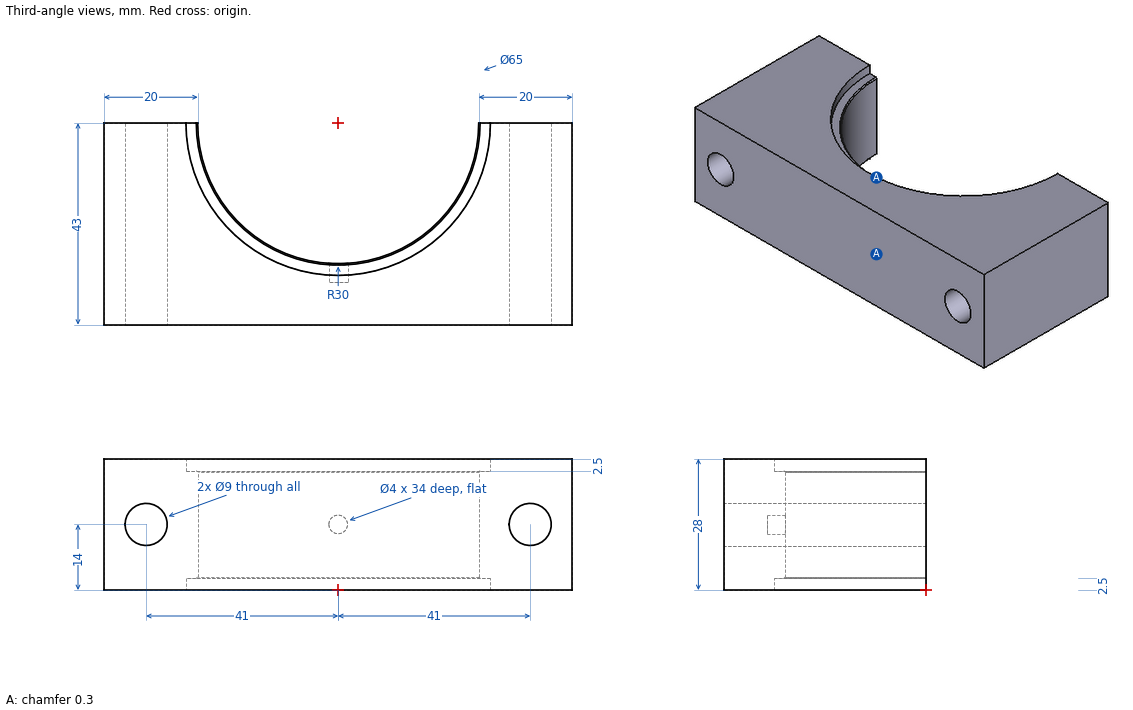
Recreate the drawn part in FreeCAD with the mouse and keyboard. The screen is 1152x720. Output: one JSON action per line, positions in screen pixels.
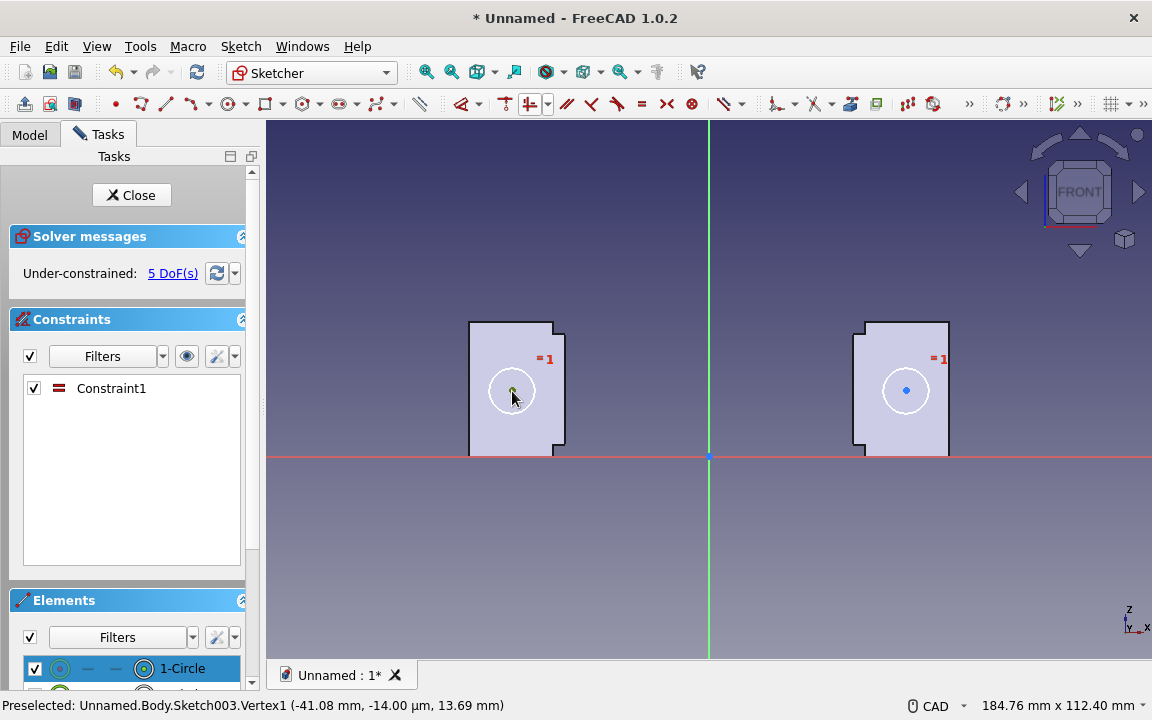
{"action": "left_click", "coordinate": [906, 391]}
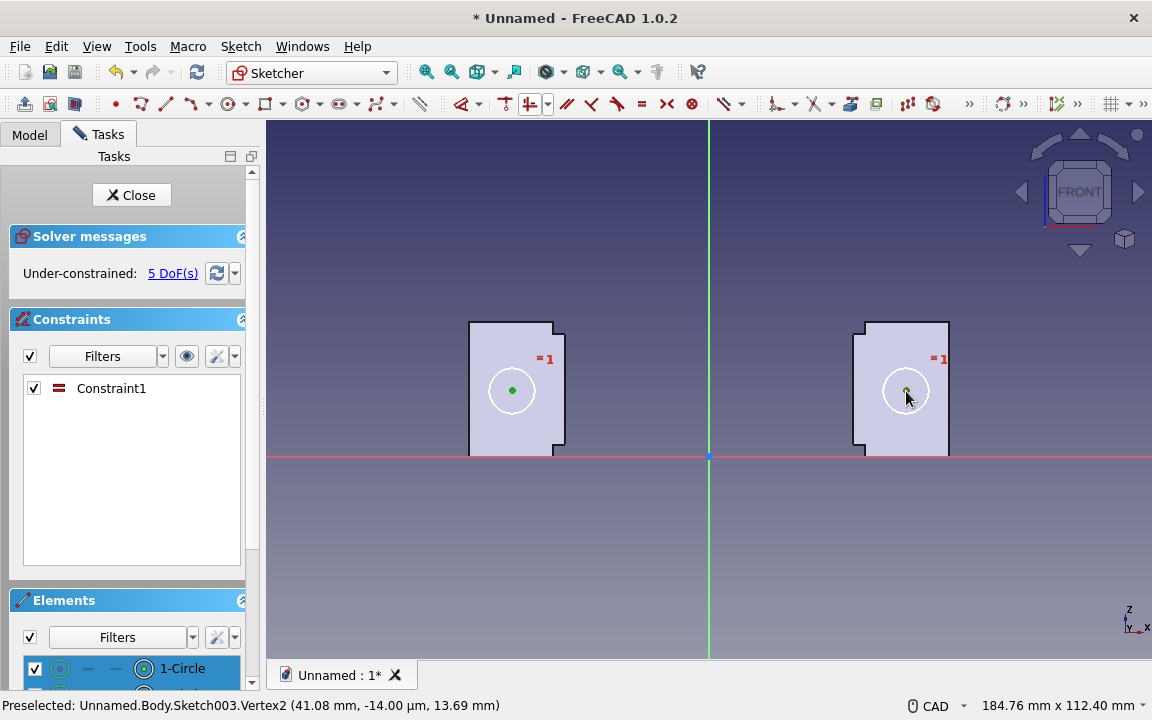
{"action": "left_click", "coordinate": [548, 104]}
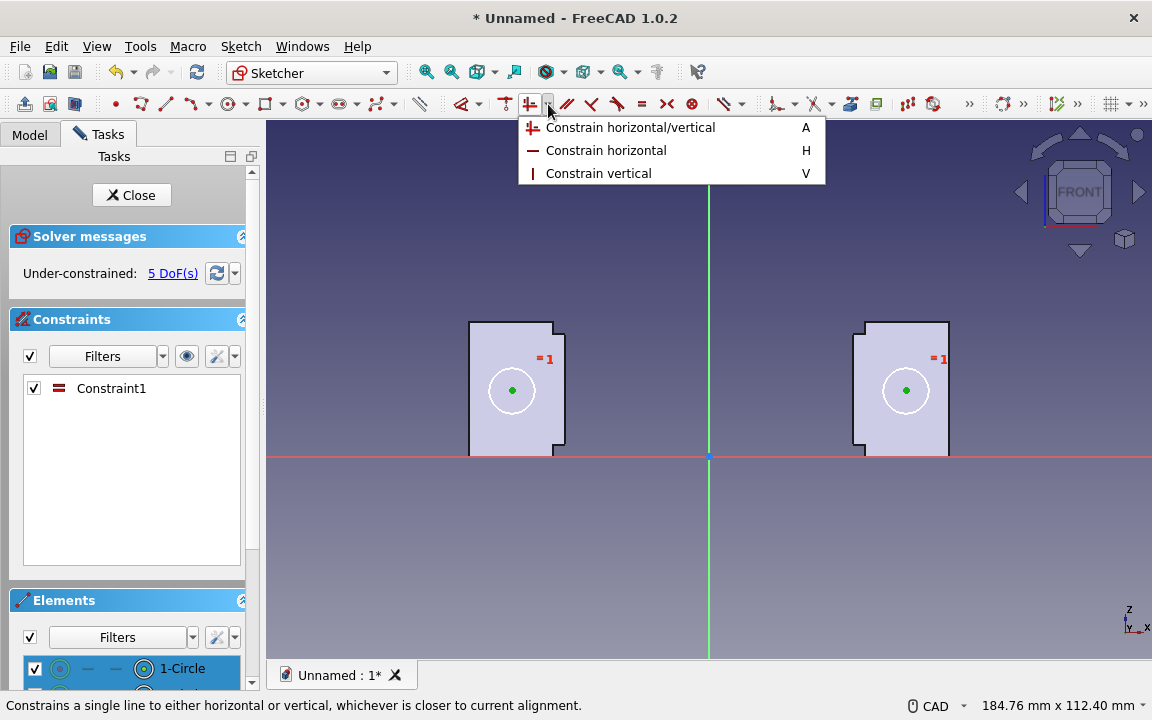
{"action": "left_click", "coordinate": [672, 150]}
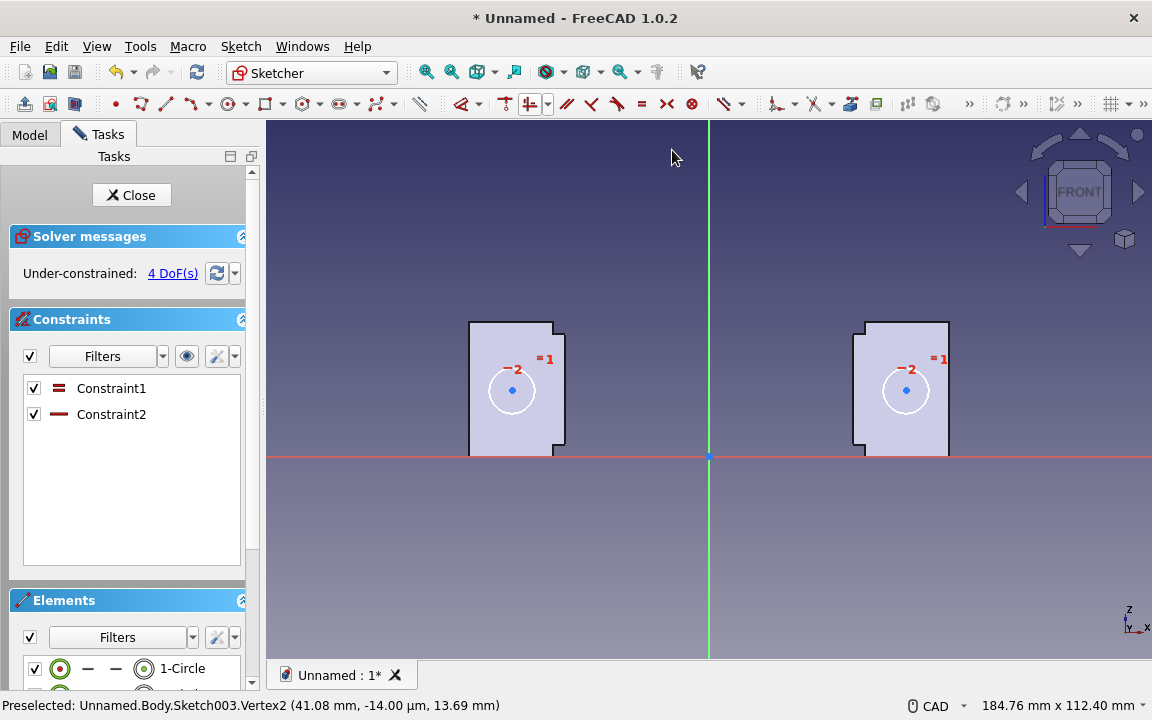
{"action": "left_click", "coordinate": [460, 104]}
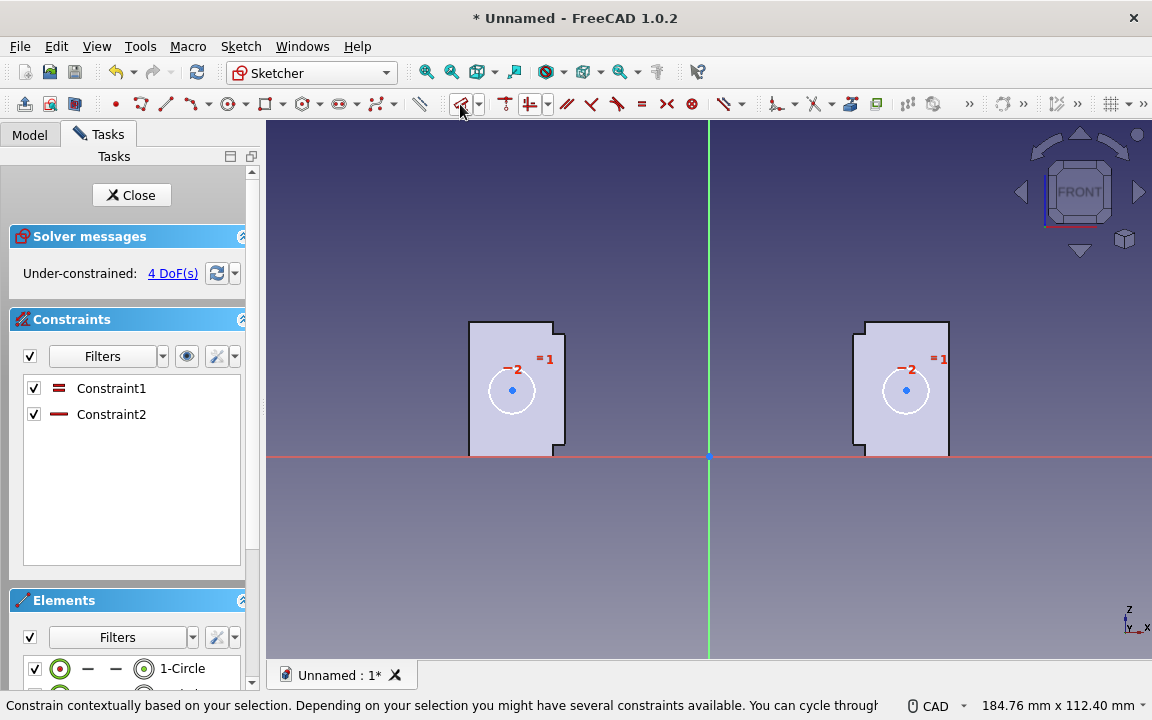
{"action": "left_click", "coordinate": [528, 375]}
{"action": "left_click", "coordinate": [551, 352]}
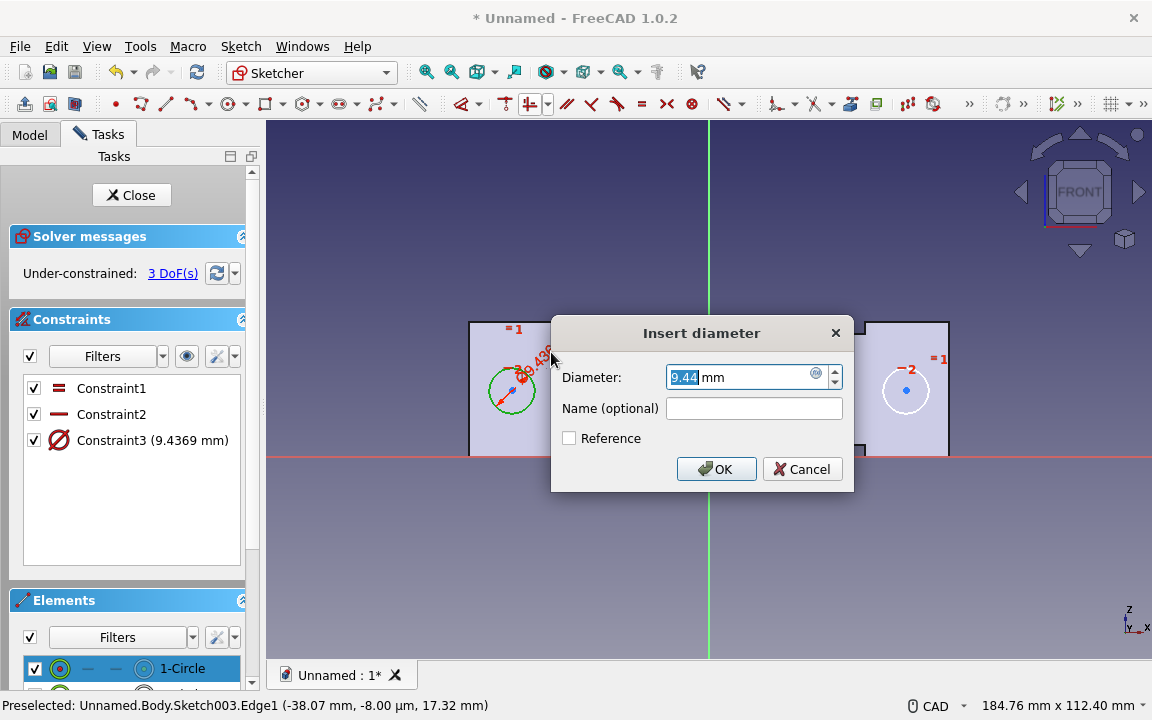
{"action": "type", "text": "9"}
{"action": "key", "text": "Return"}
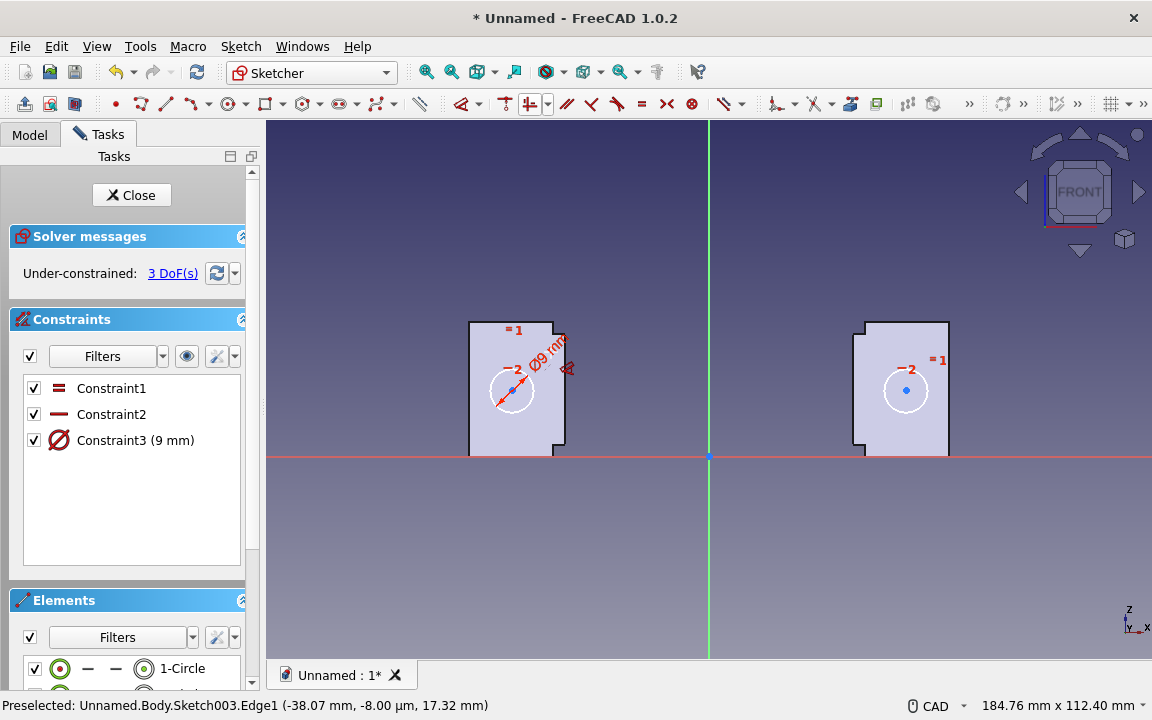
{"action": "left_click", "coordinate": [512, 391]}
{"action": "left_click", "coordinate": [611, 491]}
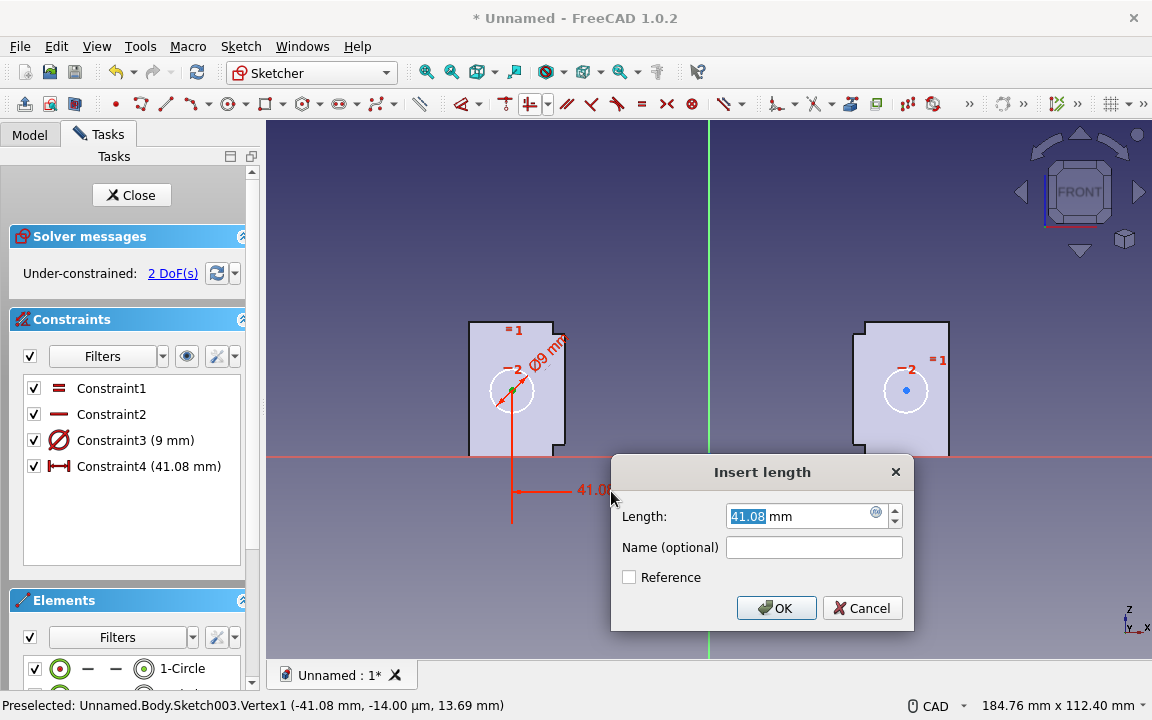
{"action": "type", "text": "41"}
{"action": "key", "text": "Return"}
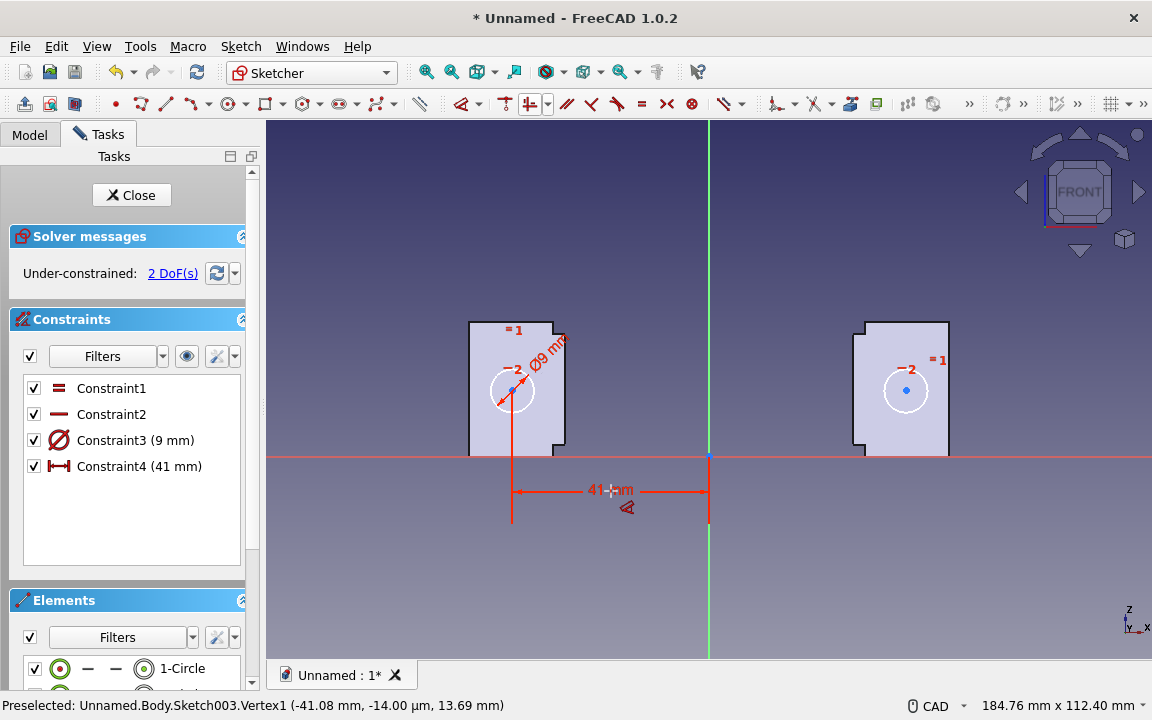
{"action": "left_click", "coordinate": [512, 391]}
{"action": "left_click", "coordinate": [478, 424]}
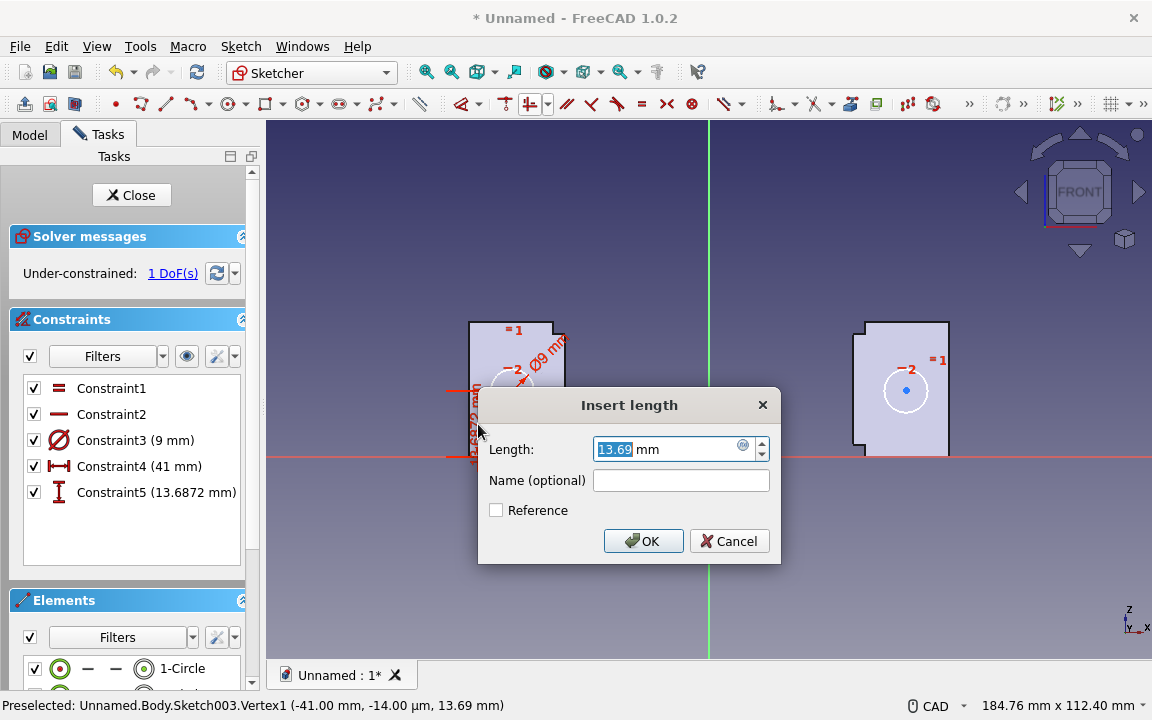
{"action": "type", "text": "14"}
{"action": "key", "text": "Return"}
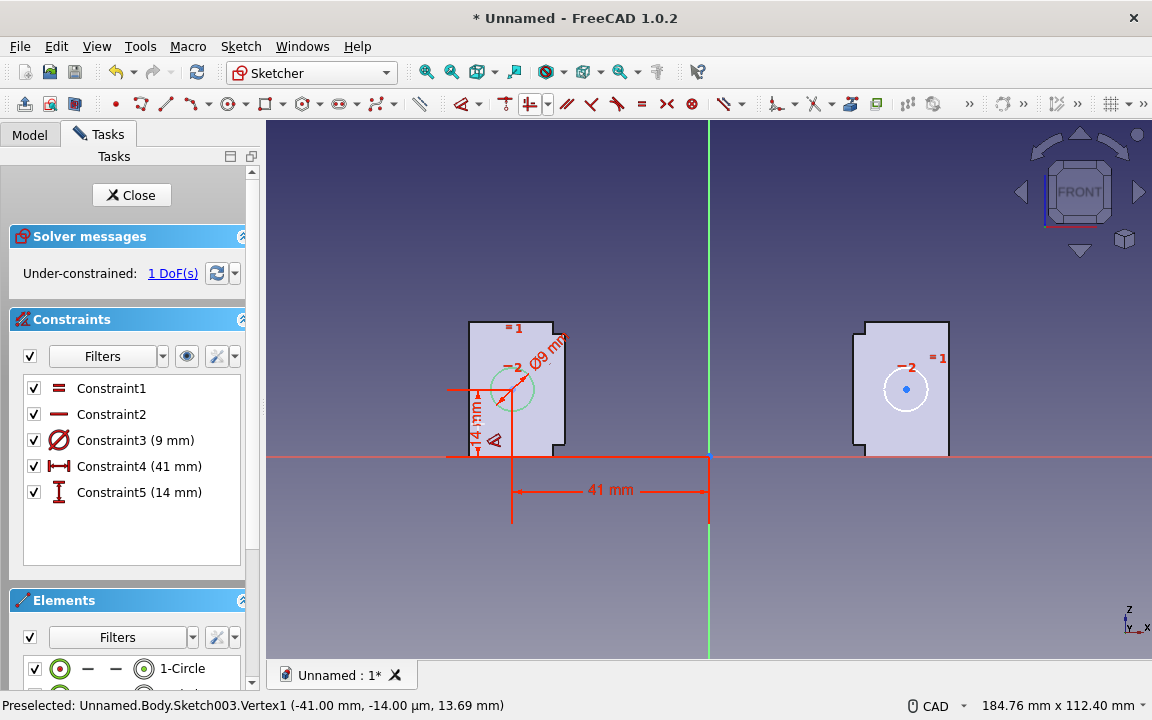
{"action": "left_click", "coordinate": [906, 390]}
{"action": "left_click", "coordinate": [807, 491]}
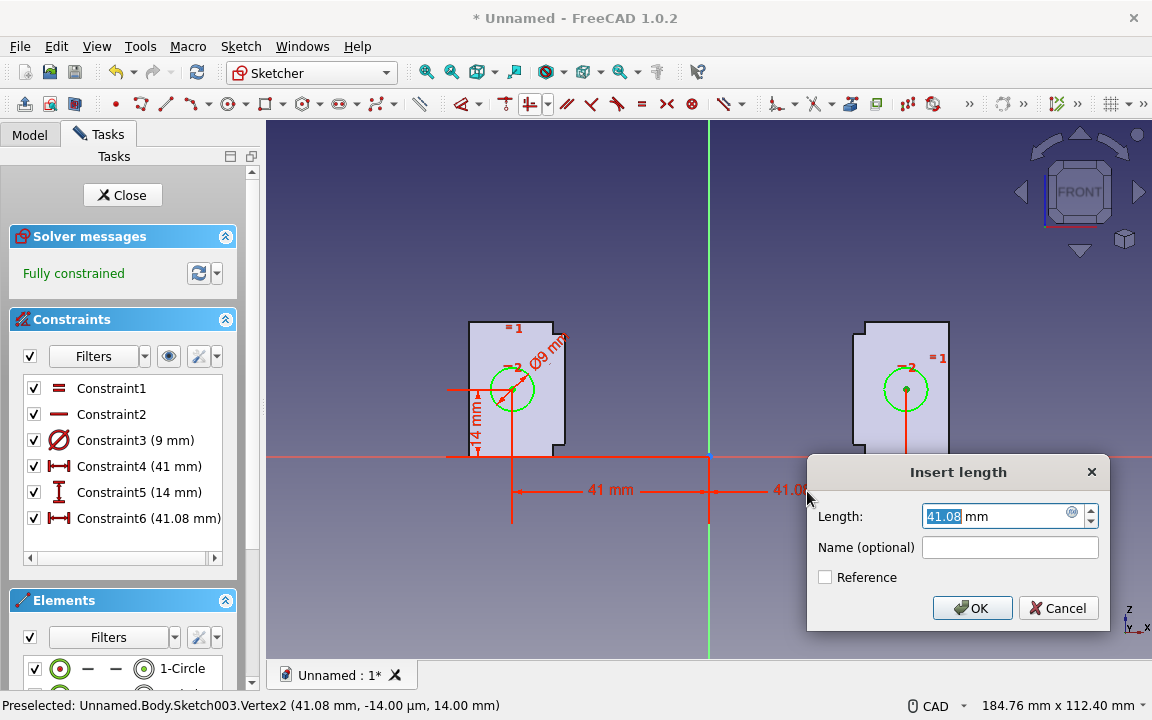
{"action": "type", "text": "41"}
{"action": "key", "text": "Return"}
{"action": "key", "text": "Escape"}